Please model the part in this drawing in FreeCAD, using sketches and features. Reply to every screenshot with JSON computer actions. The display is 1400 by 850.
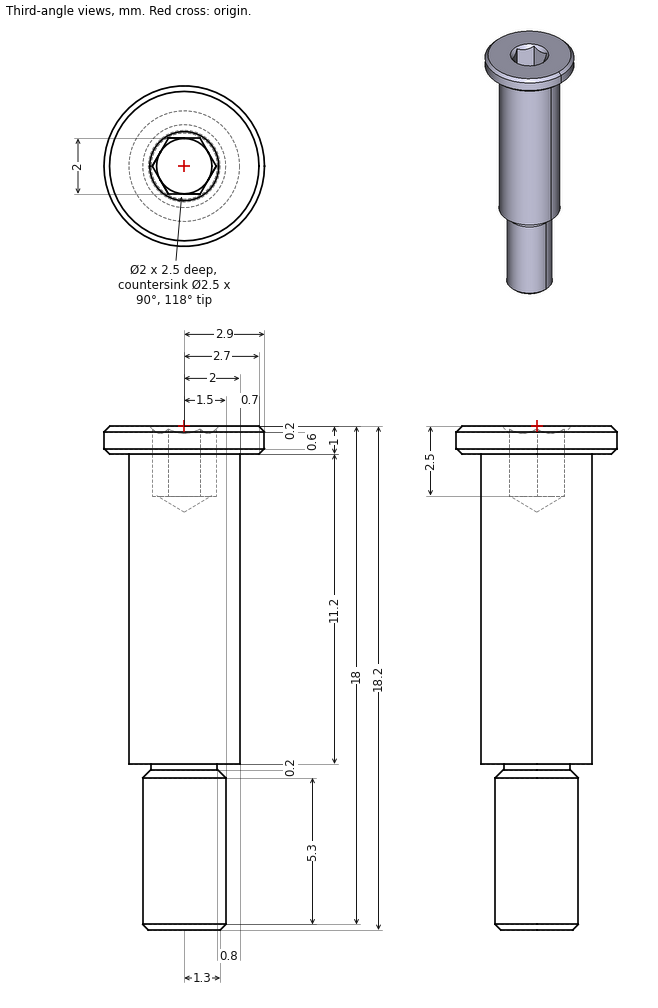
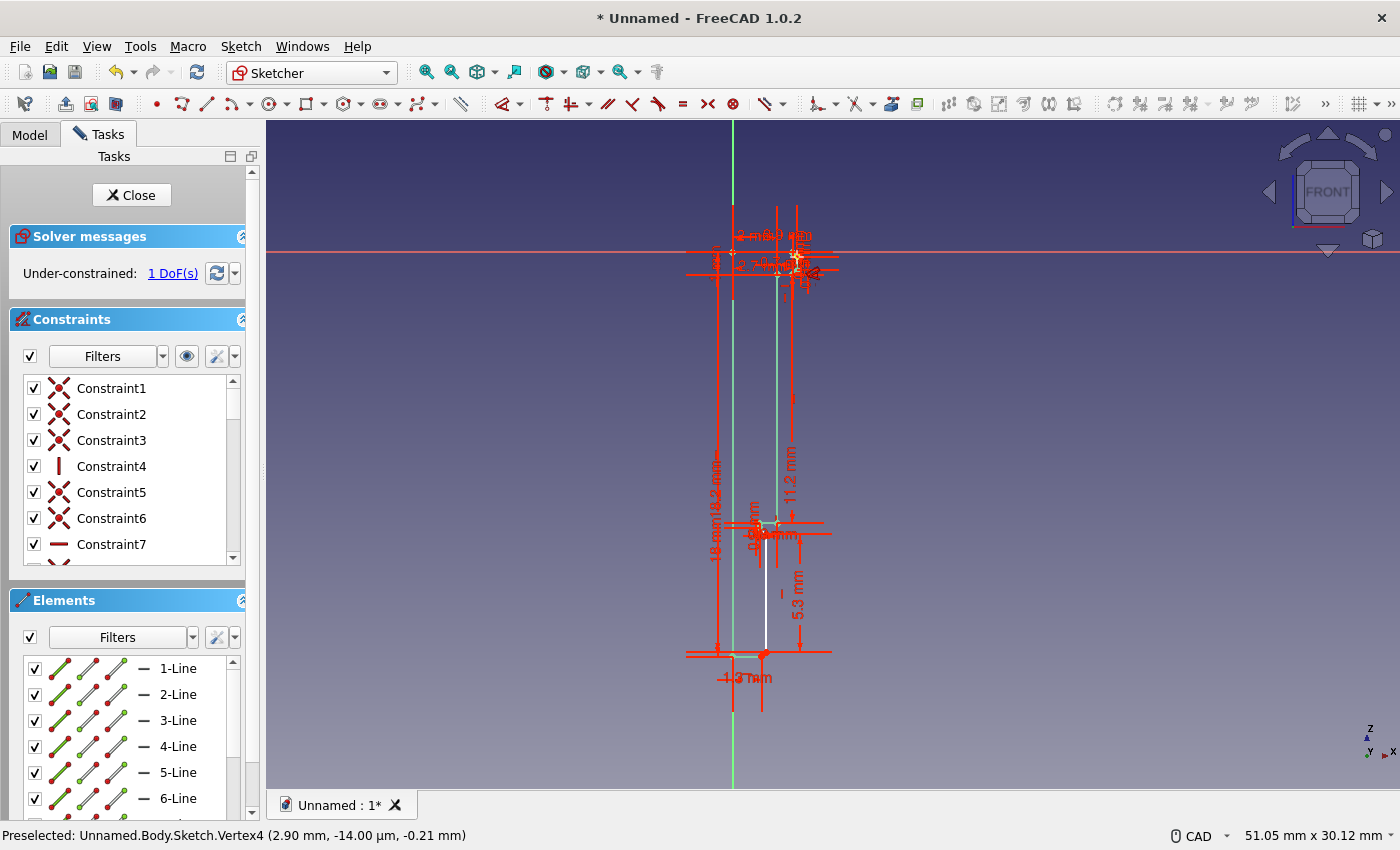
{"action": "scroll", "coordinate": [766, 534], "scroll_direction": "up", "scroll_amount": 2}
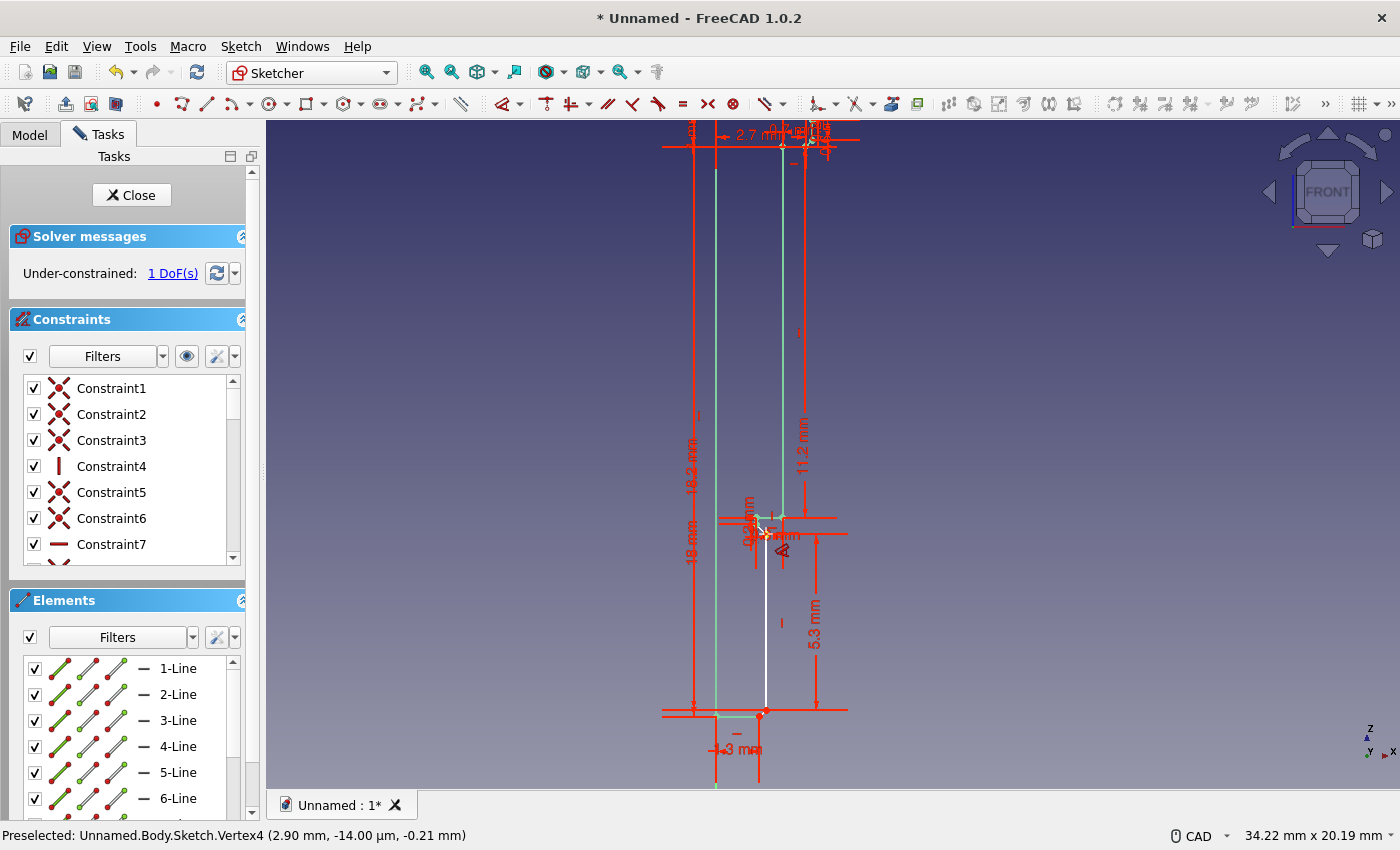
{"action": "left_click", "coordinate": [766, 534]}
{"action": "left_click", "coordinate": [741, 568]}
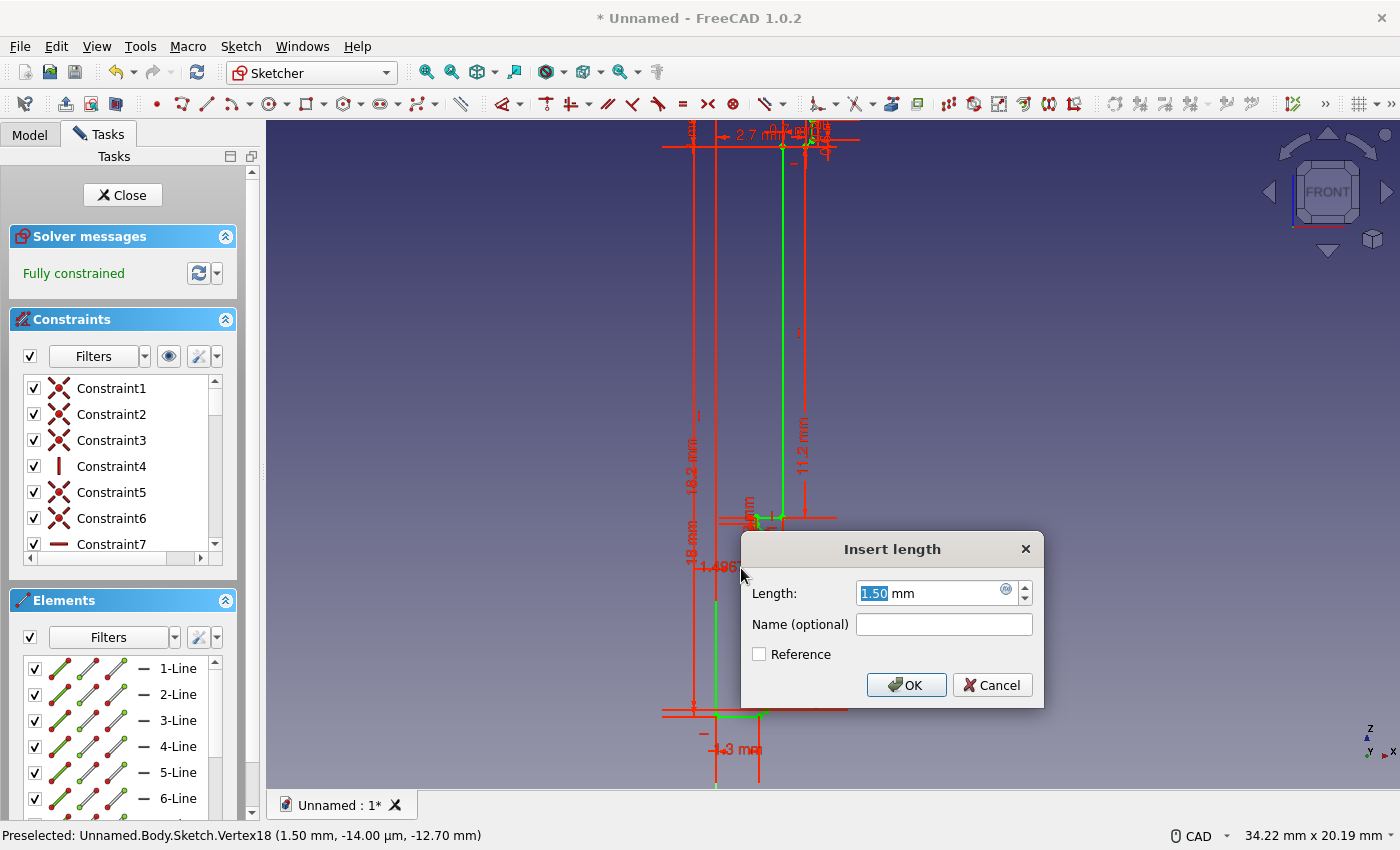
{"action": "type", "text": "1.5"}
{"action": "key", "text": "Return"}
{"action": "key", "text": "Escape"}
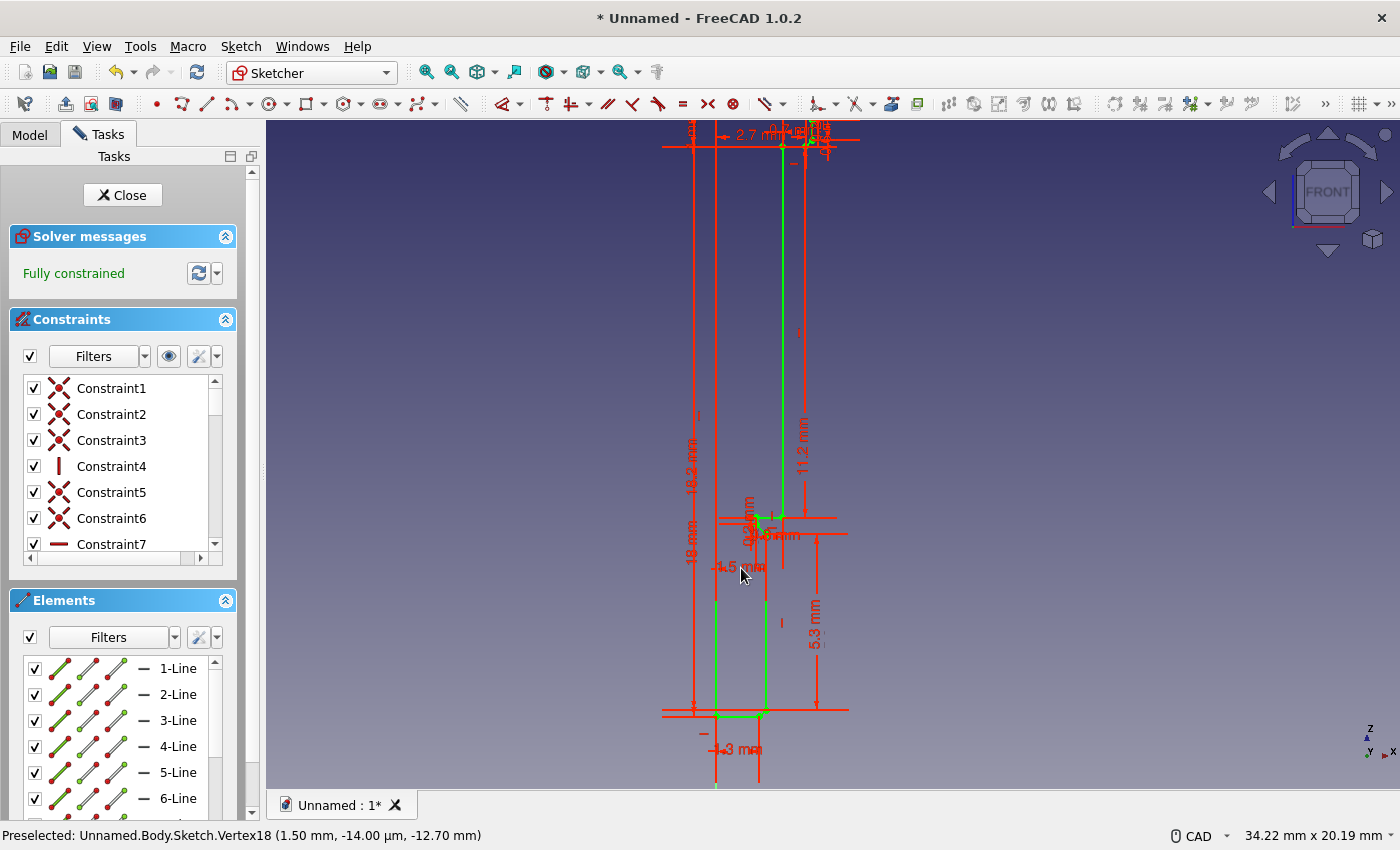
{"action": "left_click", "coordinate": [123, 195]}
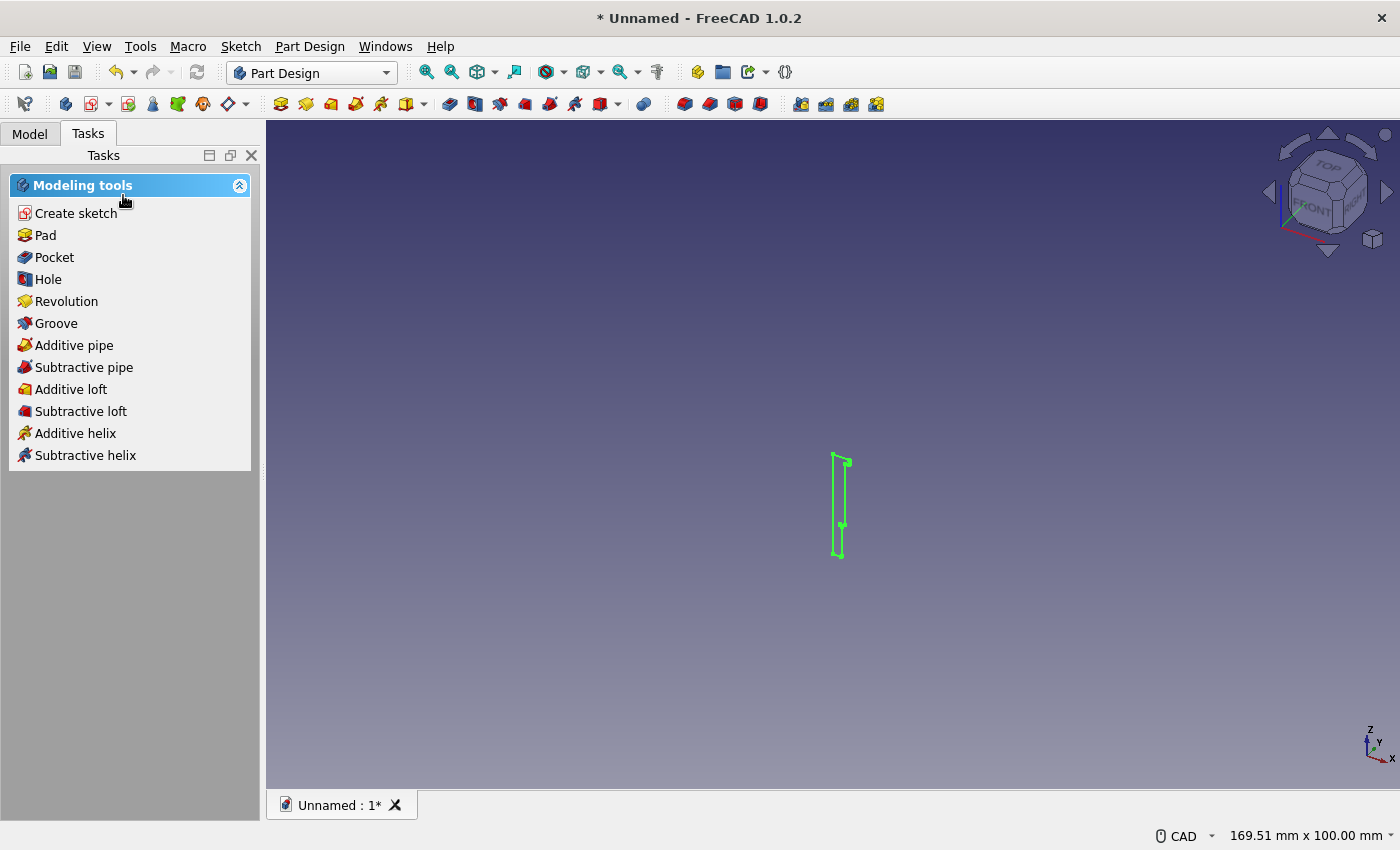
{"action": "left_click", "coordinate": [306, 104]}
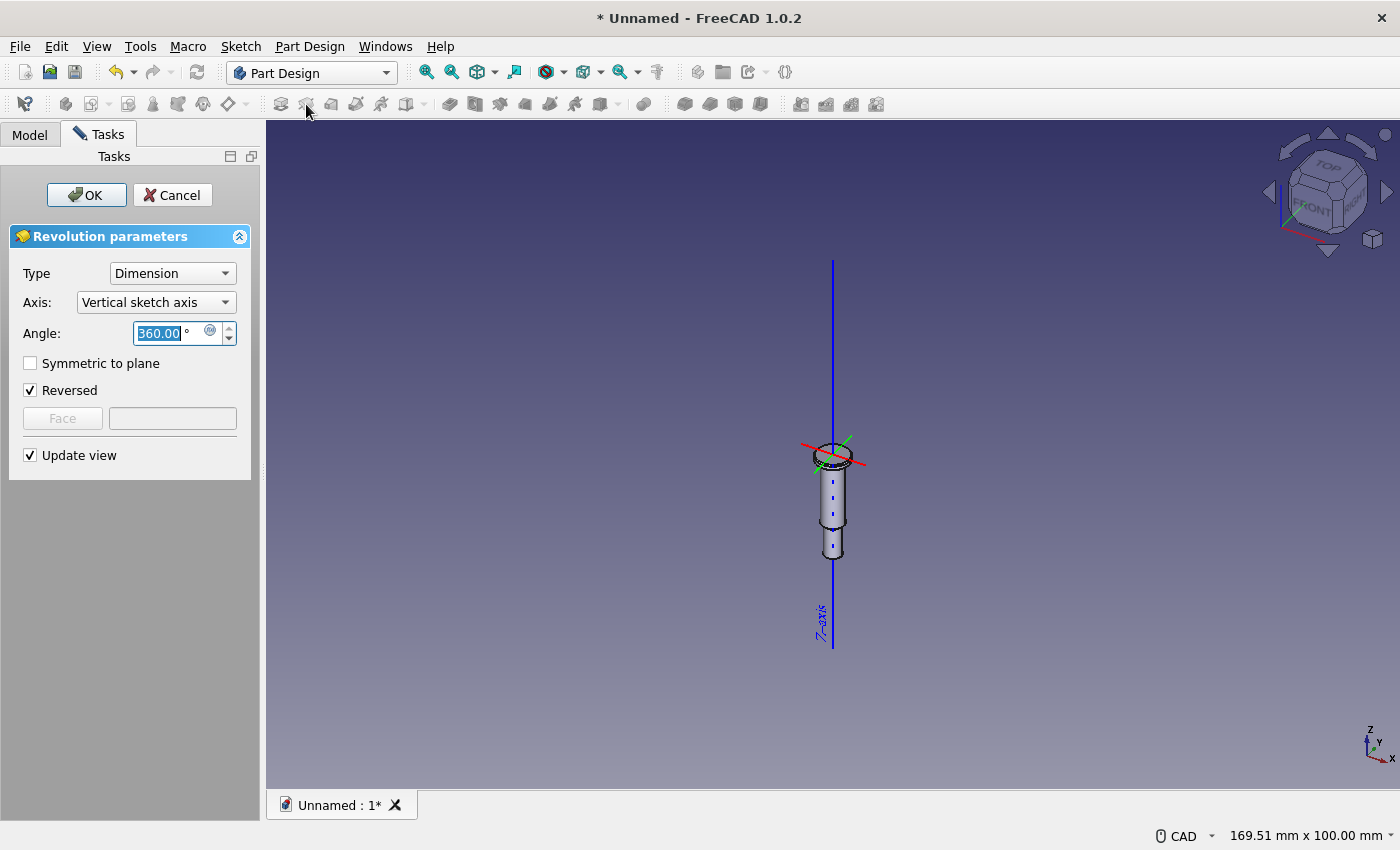
{"action": "left_click", "coordinate": [87, 195]}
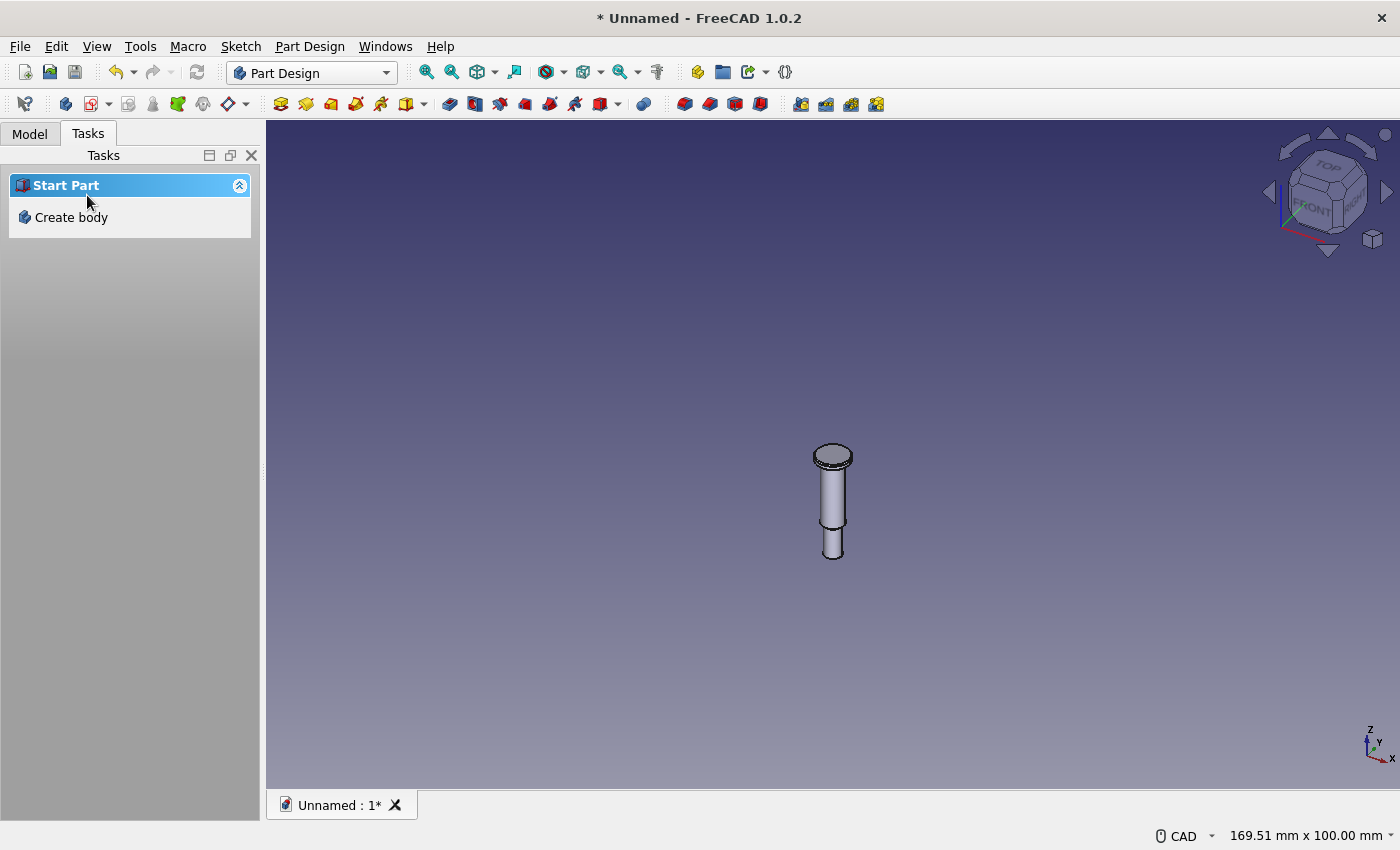
{"action": "left_click", "coordinate": [427, 72]}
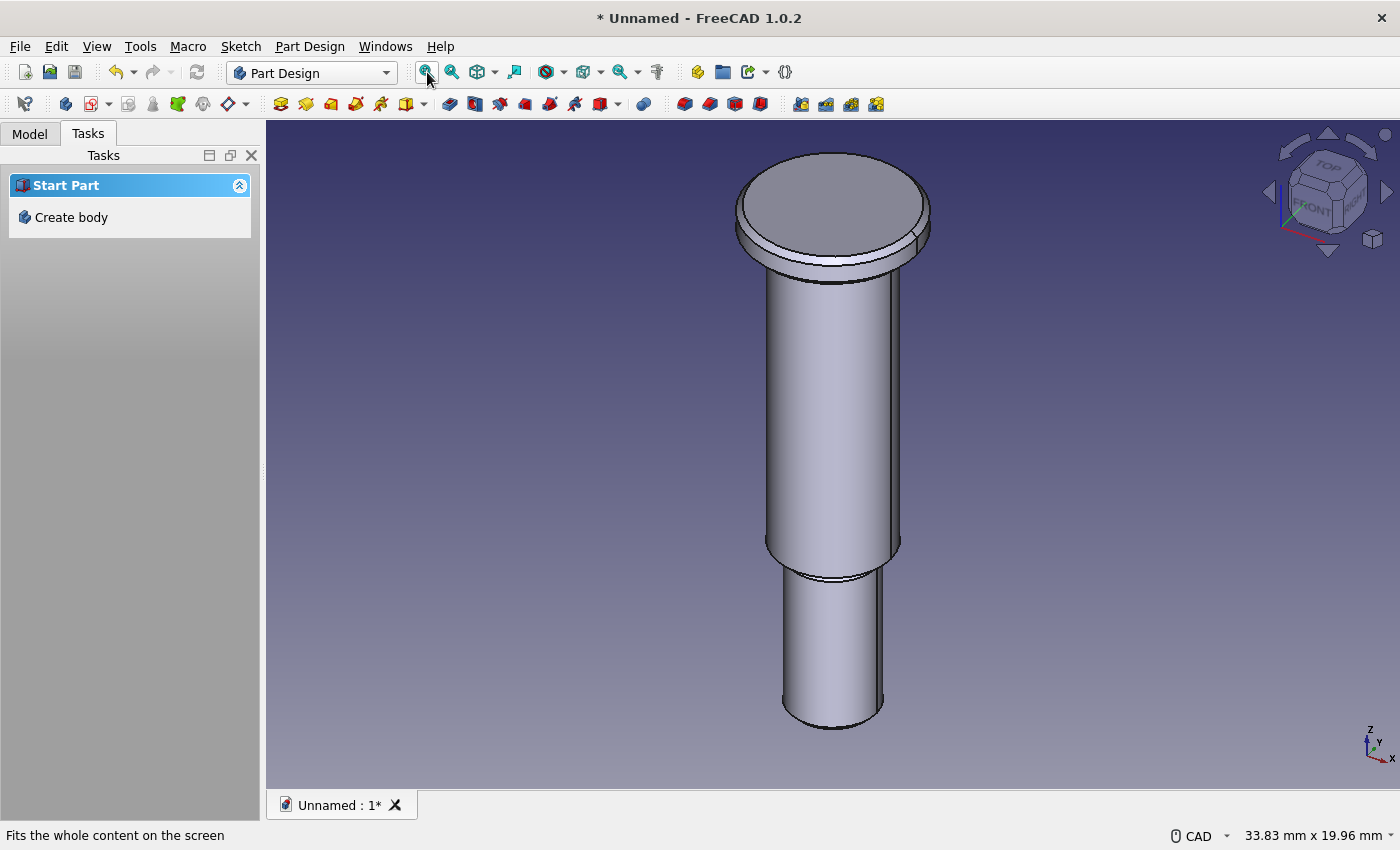
{"action": "left_click", "coordinate": [90, 104]}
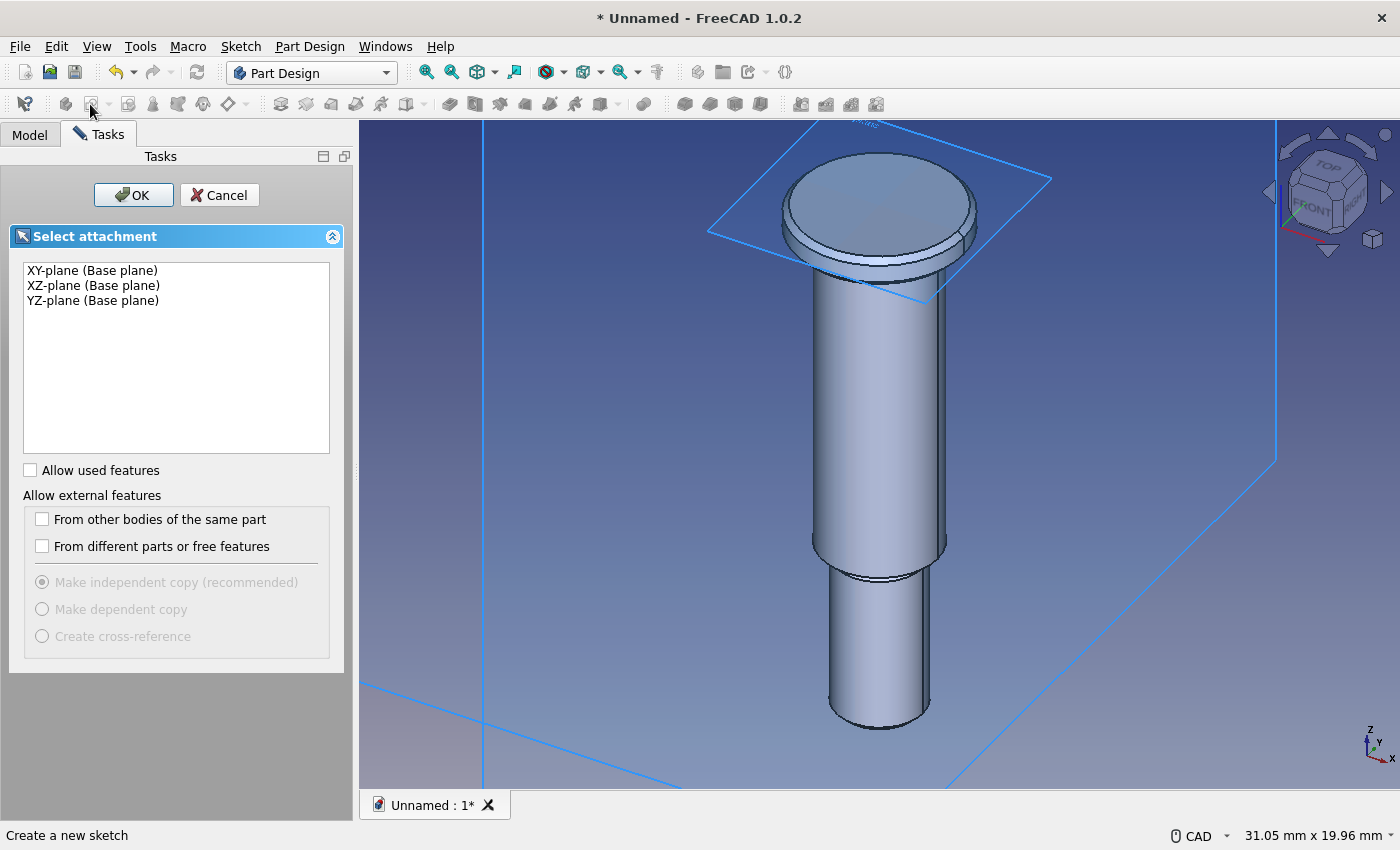
{"action": "left_click", "coordinate": [84, 270]}